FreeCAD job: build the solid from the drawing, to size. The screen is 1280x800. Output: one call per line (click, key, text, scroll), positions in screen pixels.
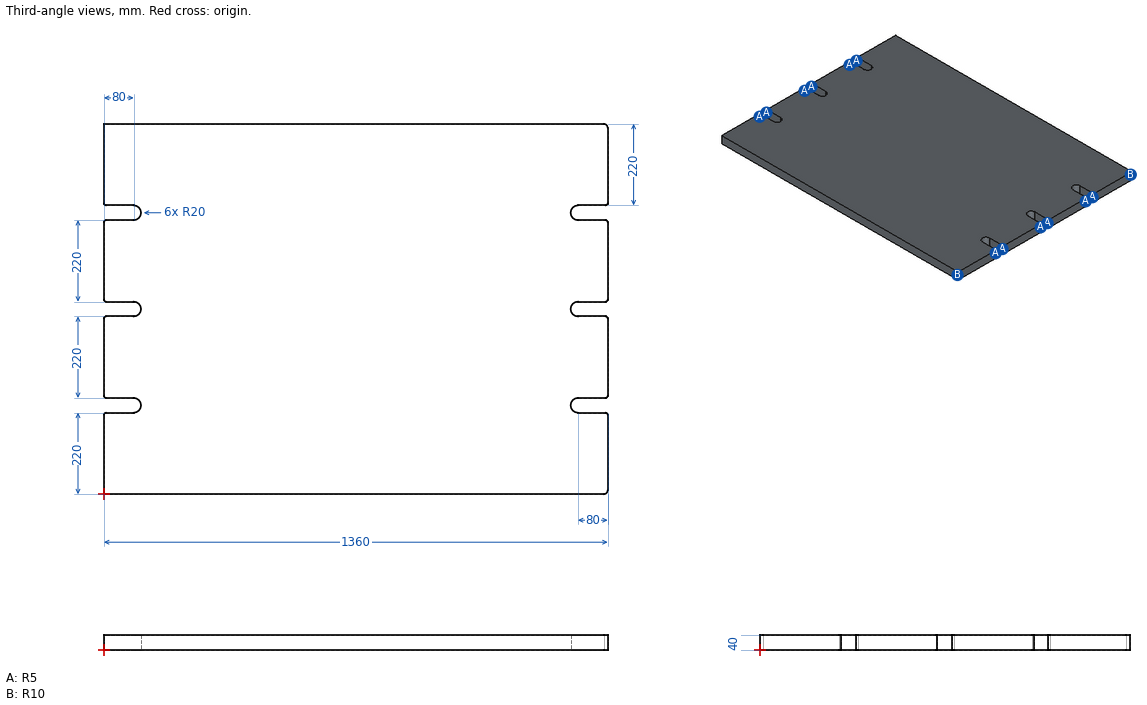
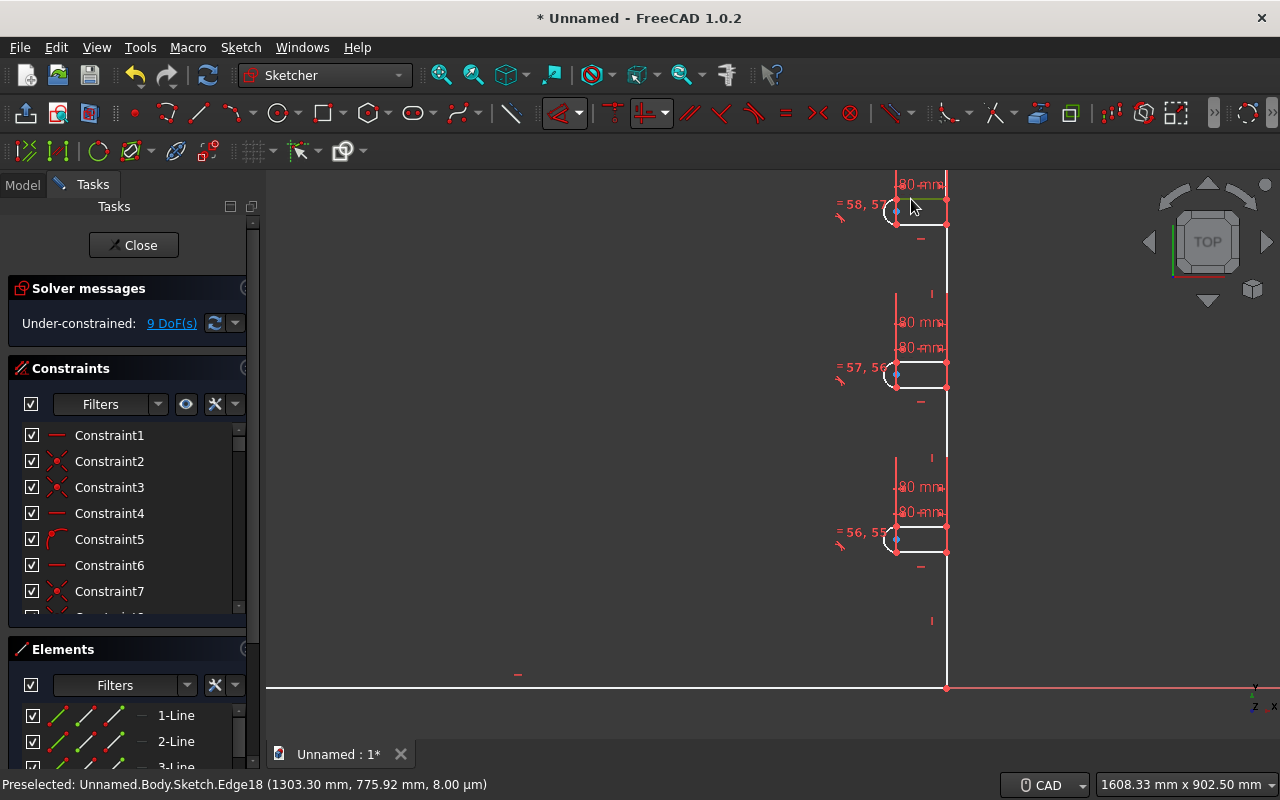
click(582, 114)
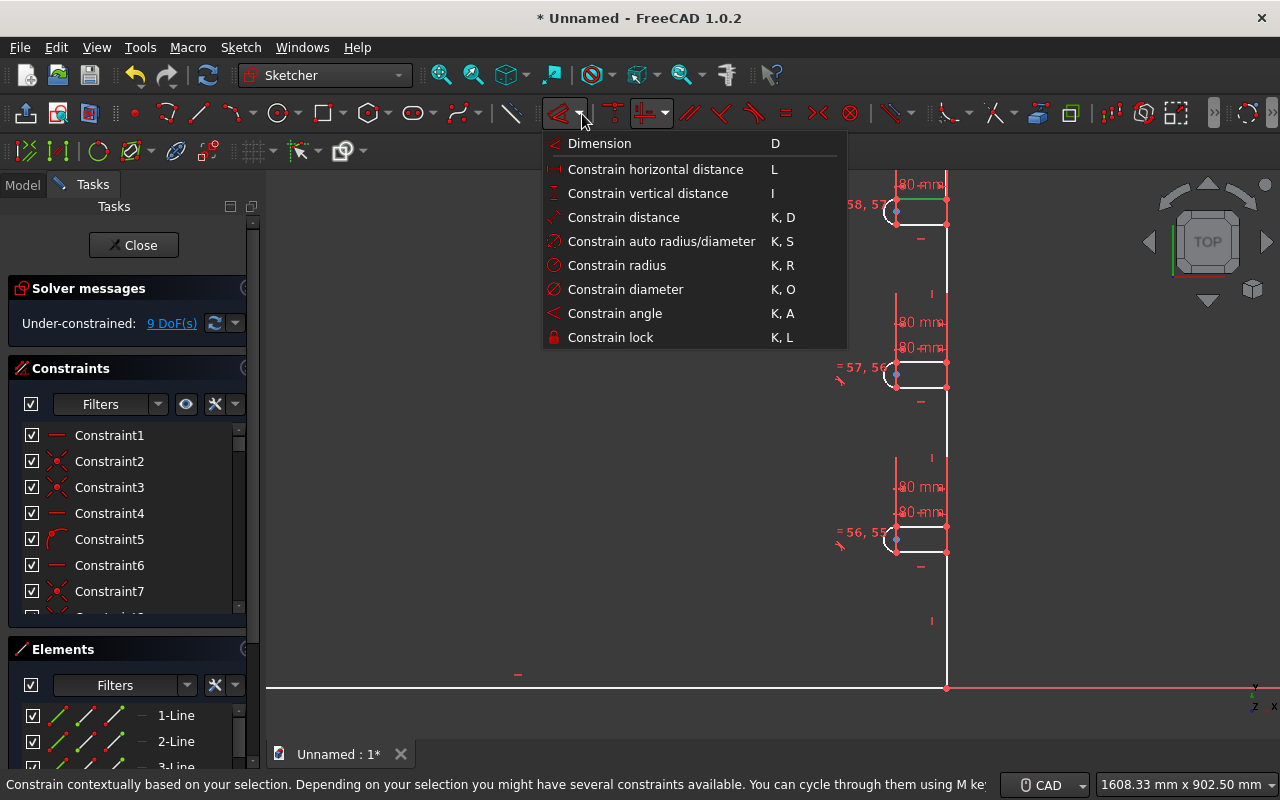
click(695, 169)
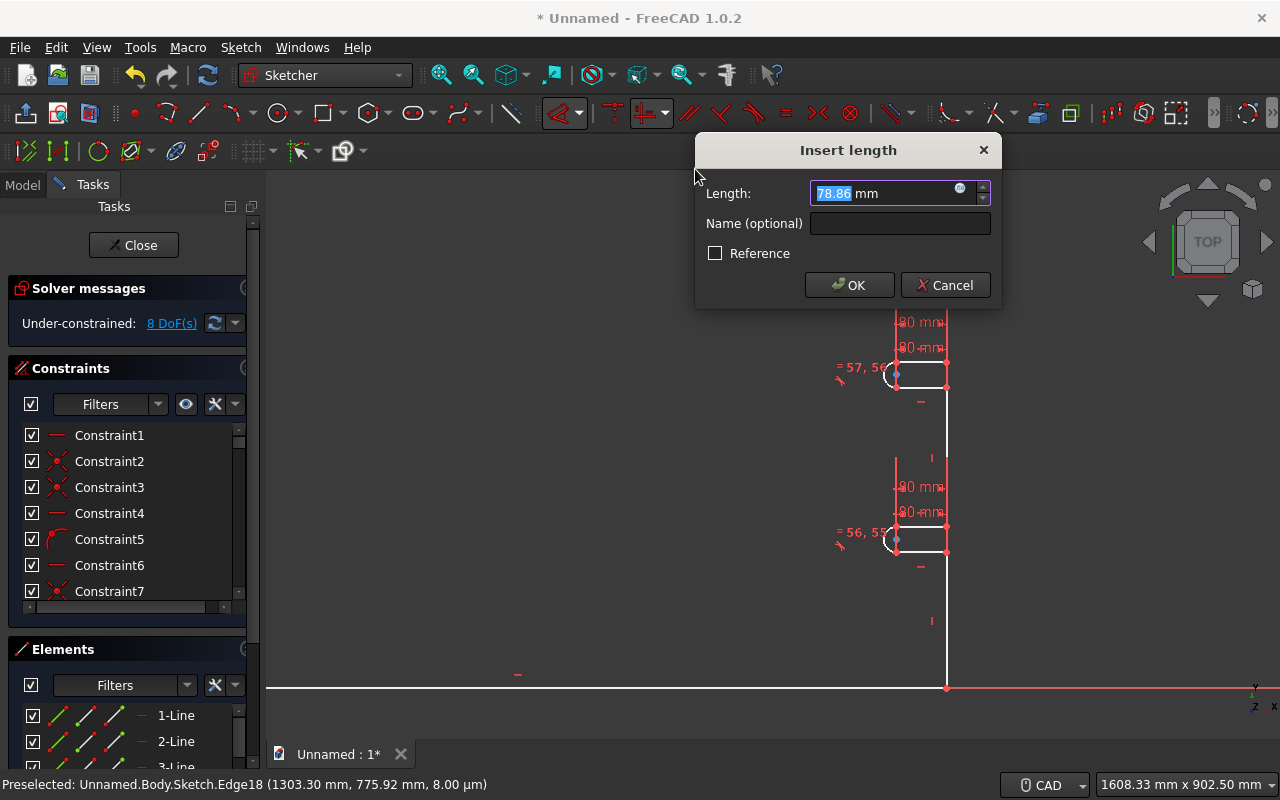
text(80)
key(Return)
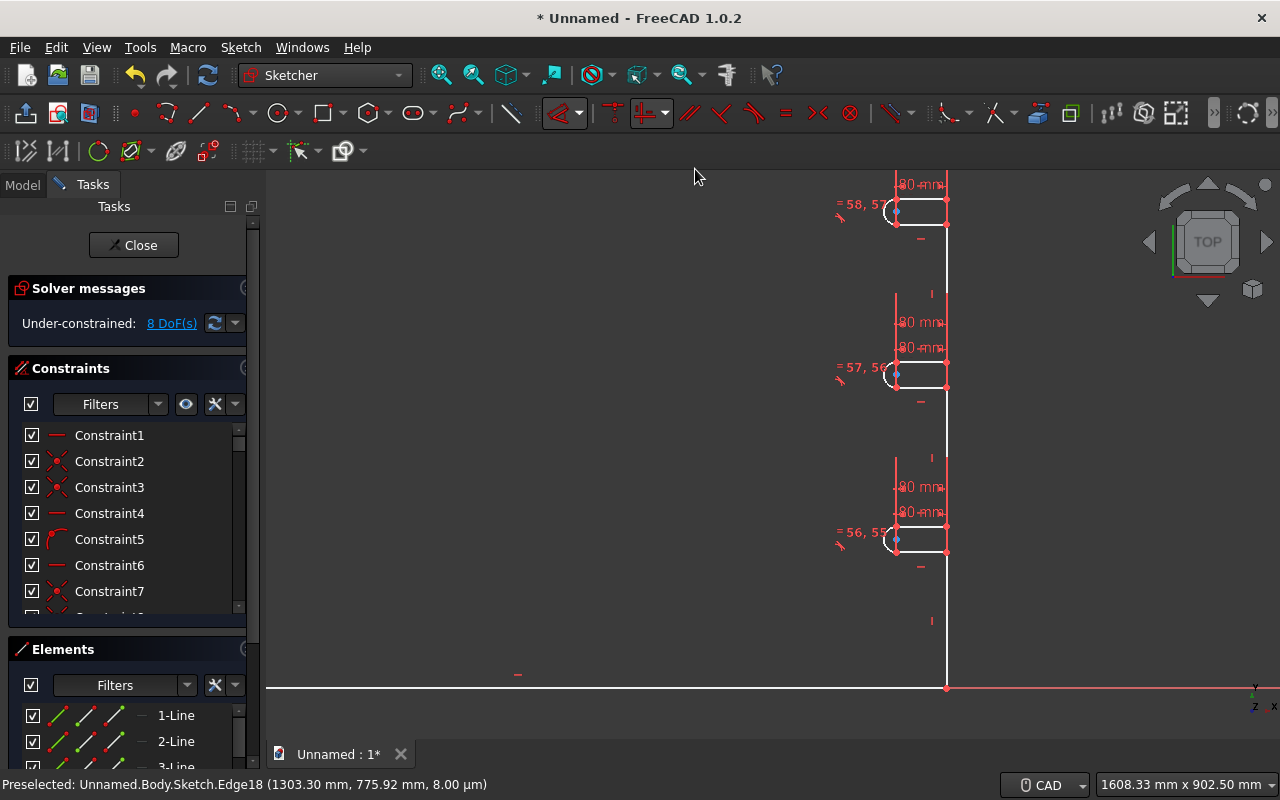
scroll(931, 553, down, 3)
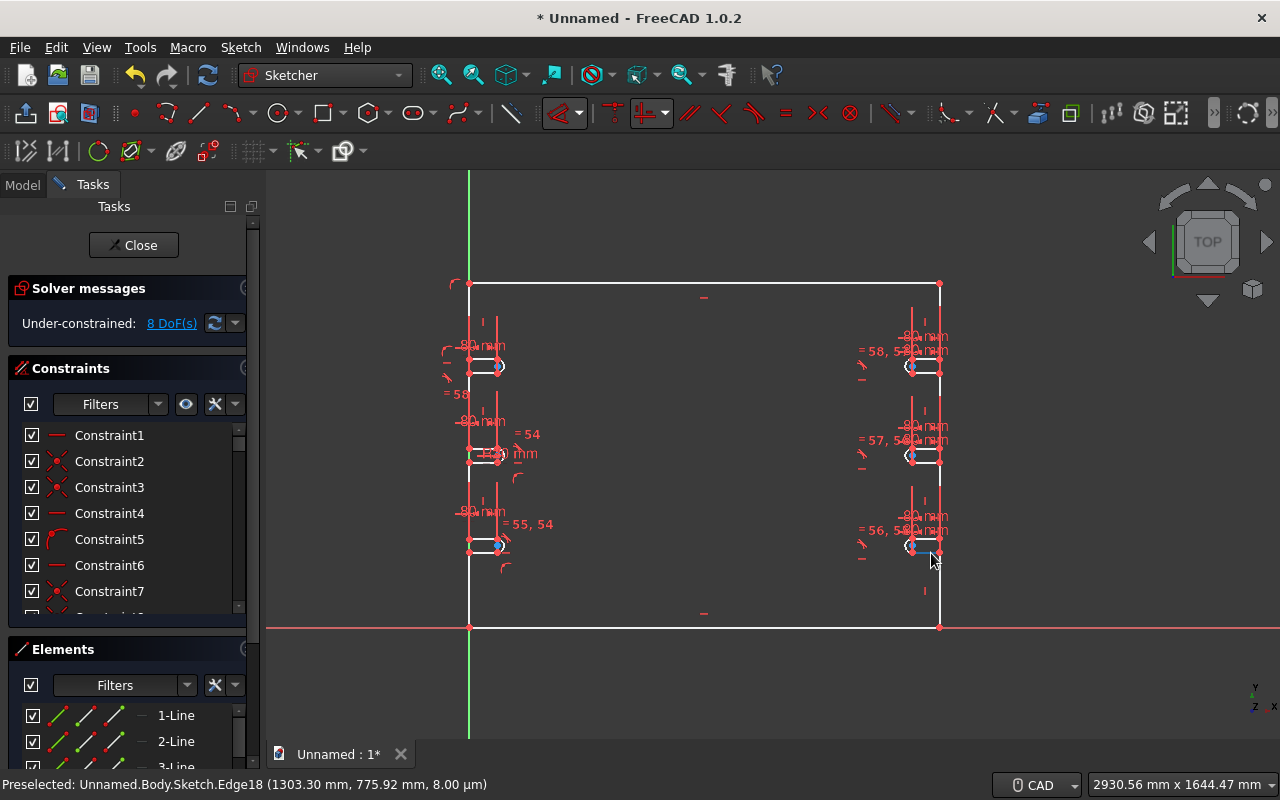
click(469, 403)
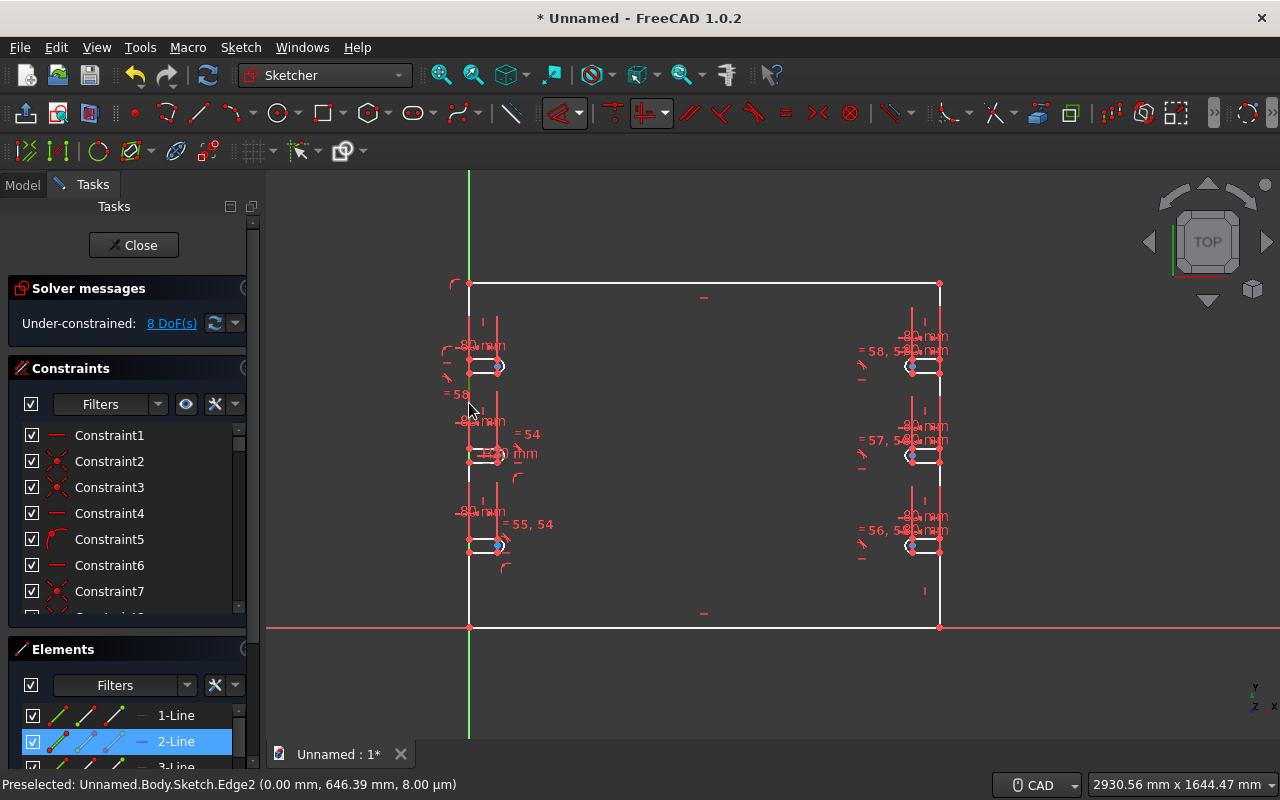
click(582, 114)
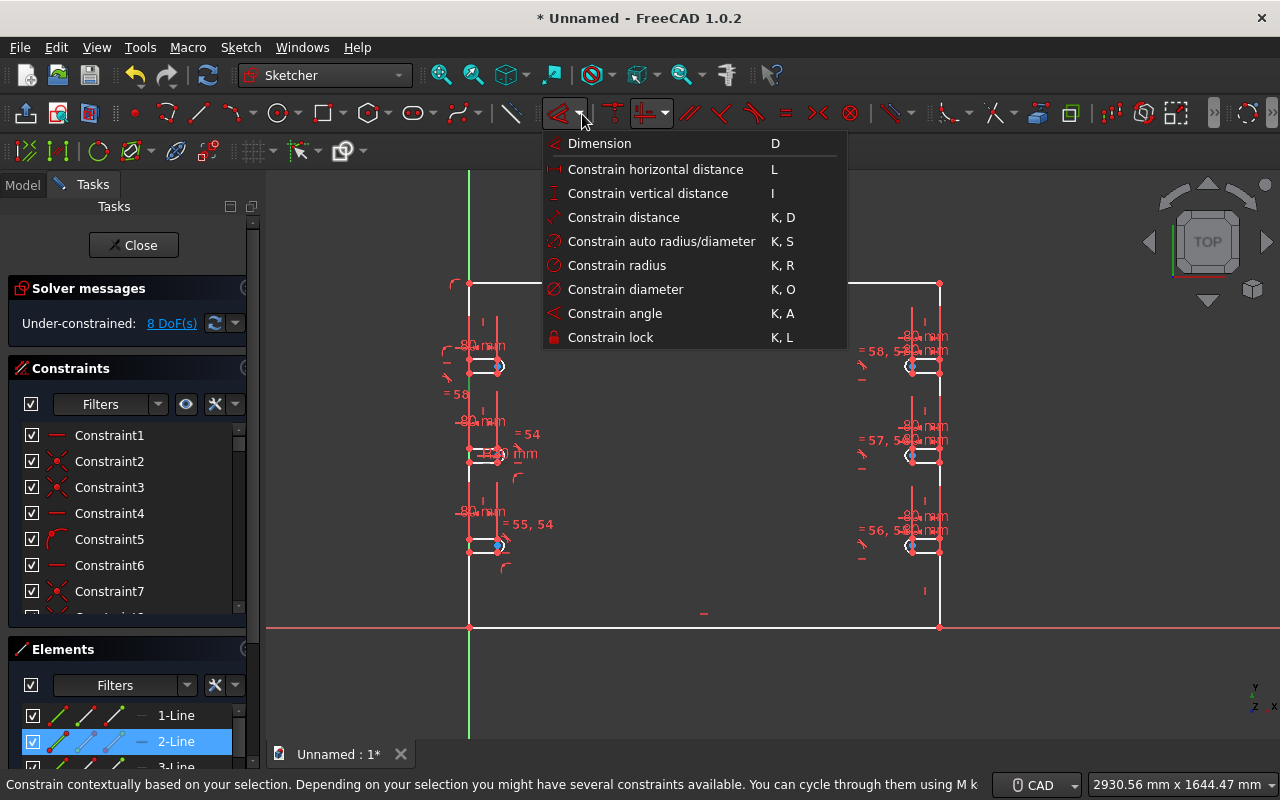
click(695, 193)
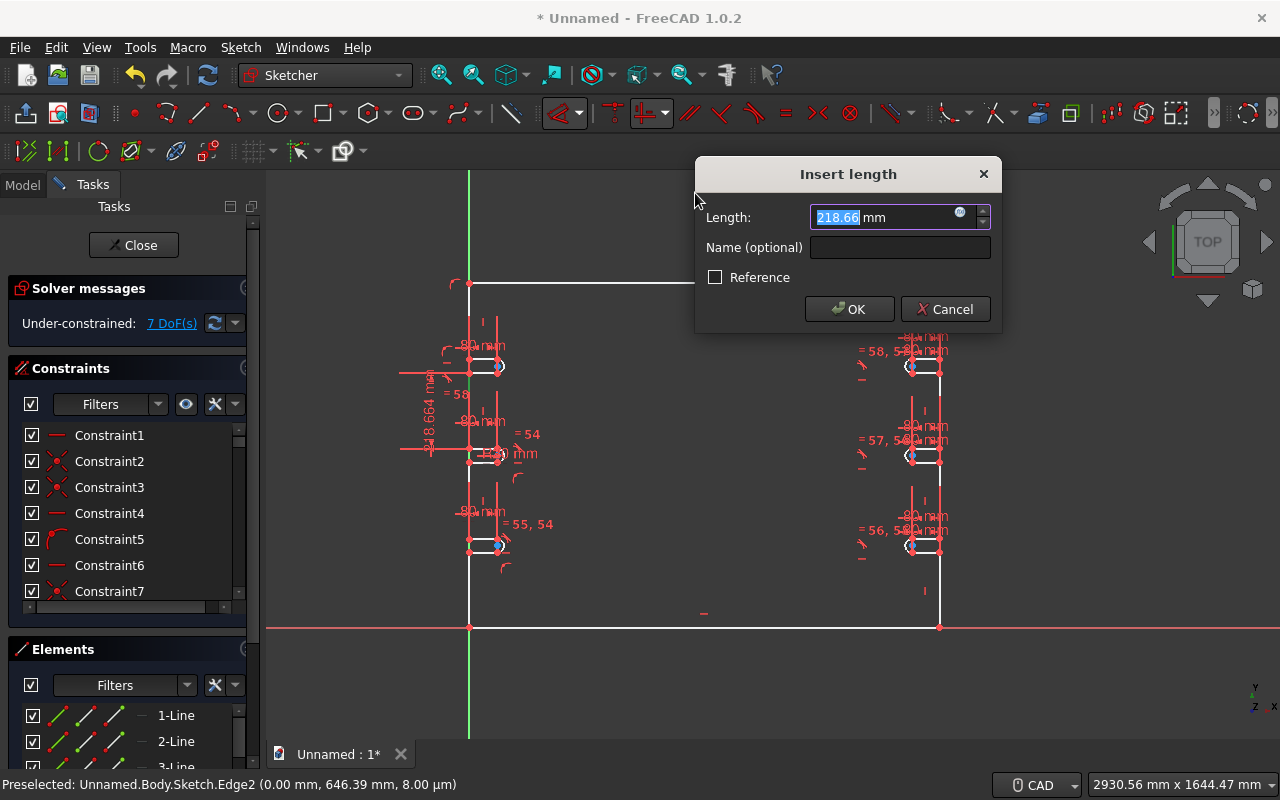
text(220)
key(Return)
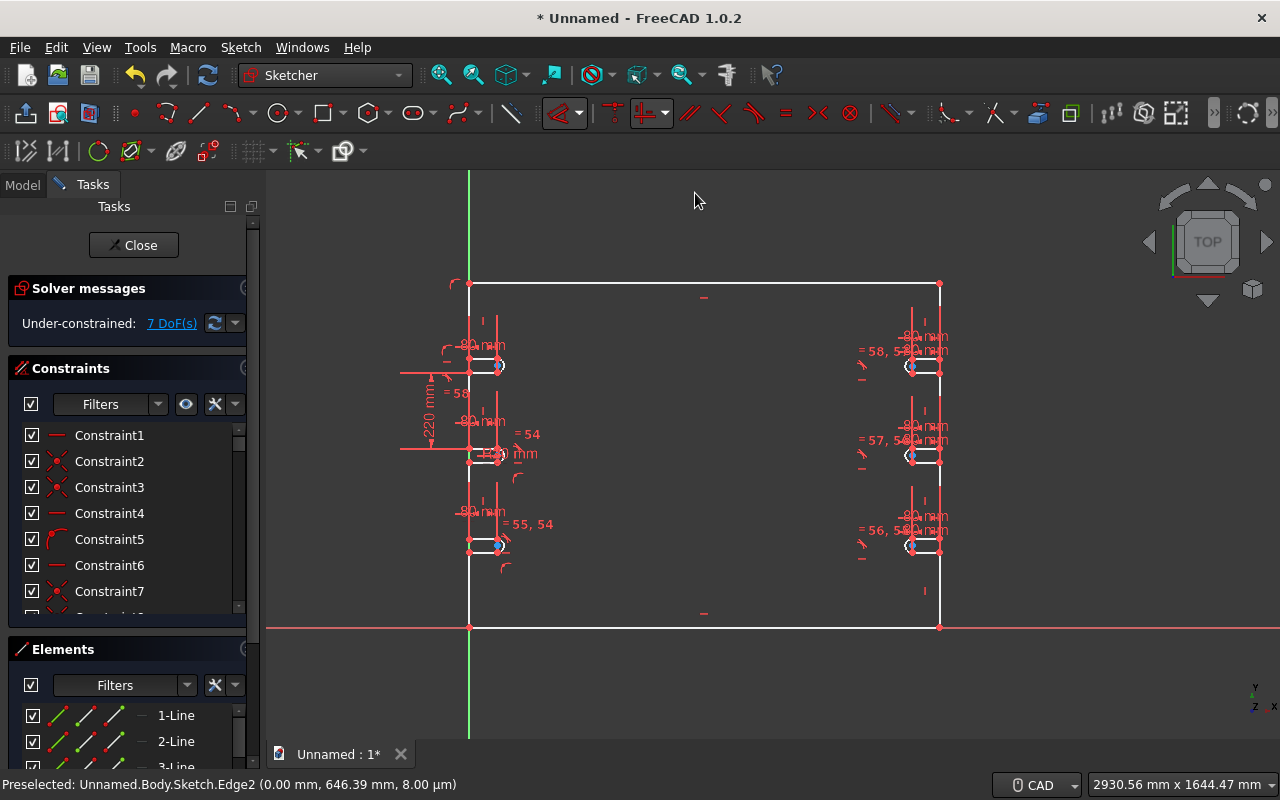
click(469, 485)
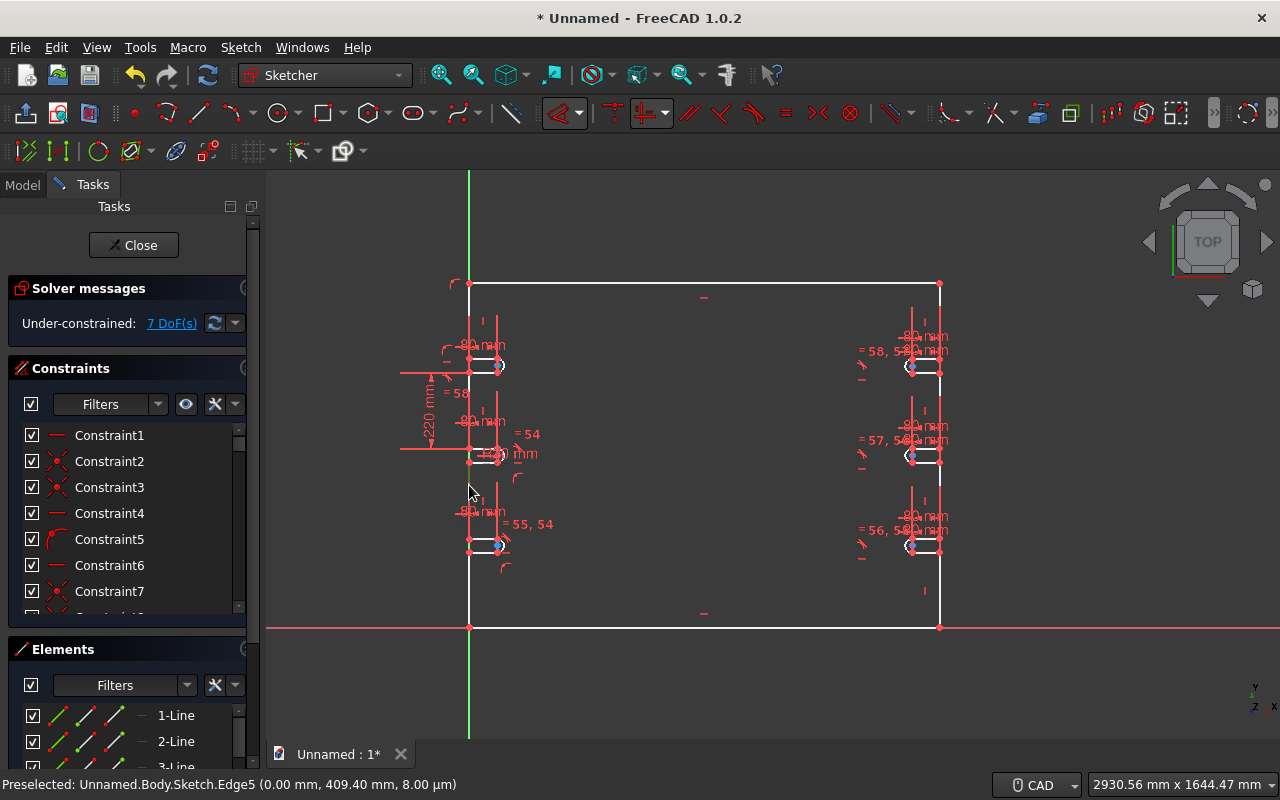
click(582, 114)